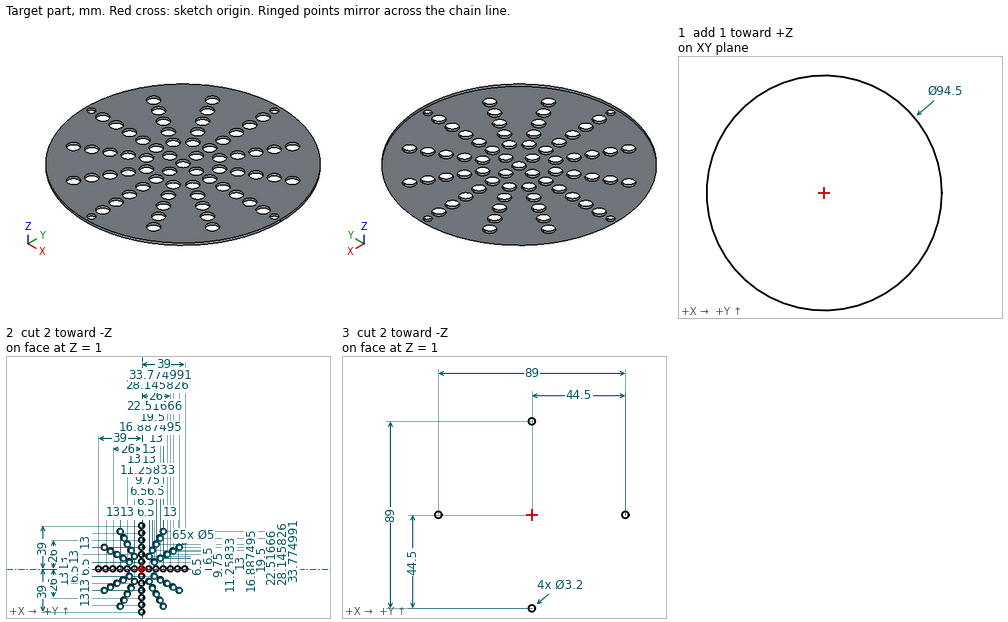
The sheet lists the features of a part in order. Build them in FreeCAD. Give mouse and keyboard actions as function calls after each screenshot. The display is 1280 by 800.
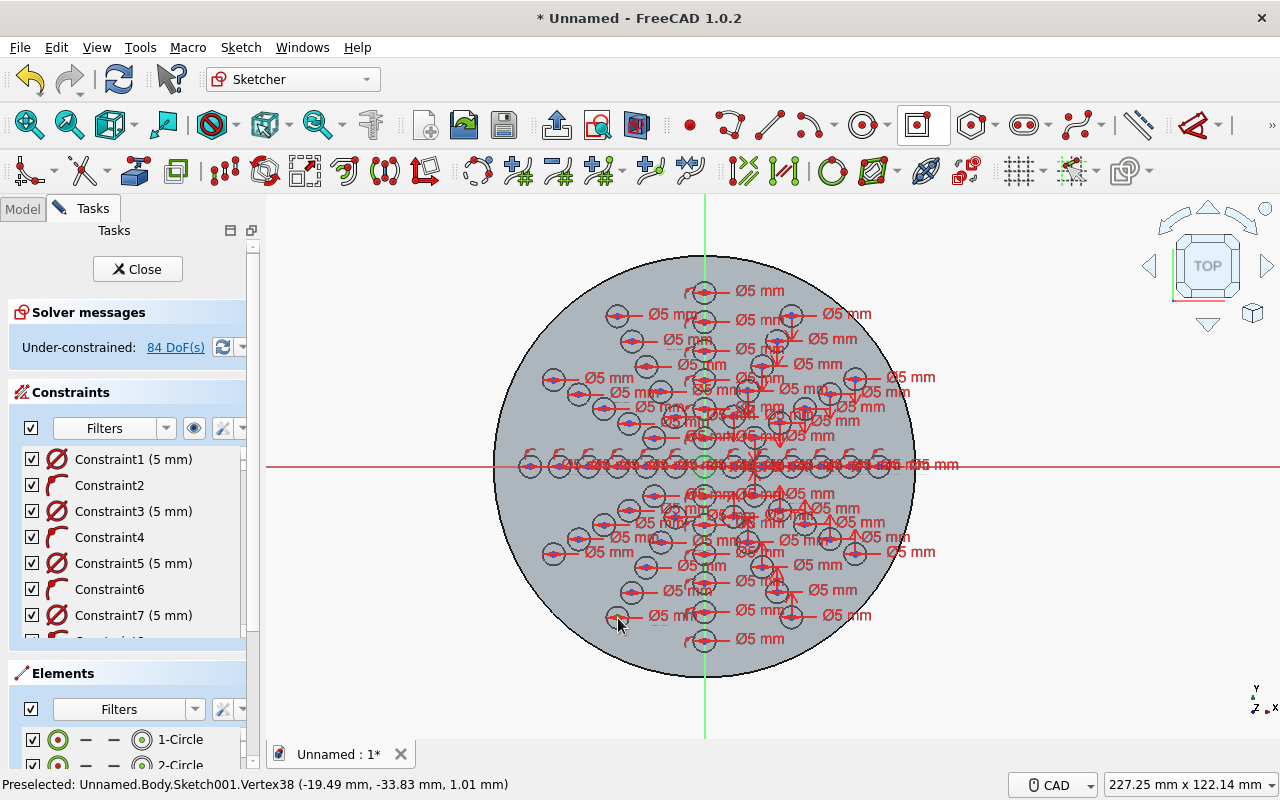
click(705, 257)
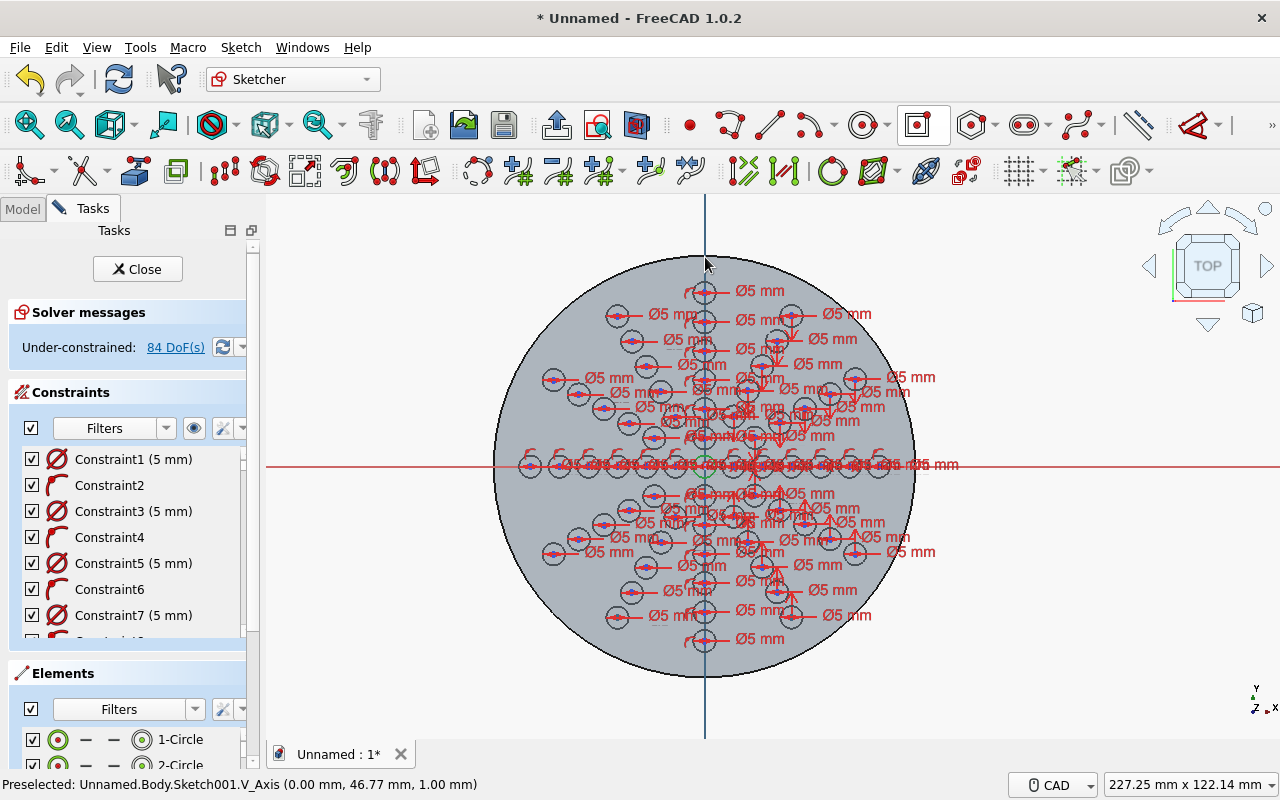
key(s)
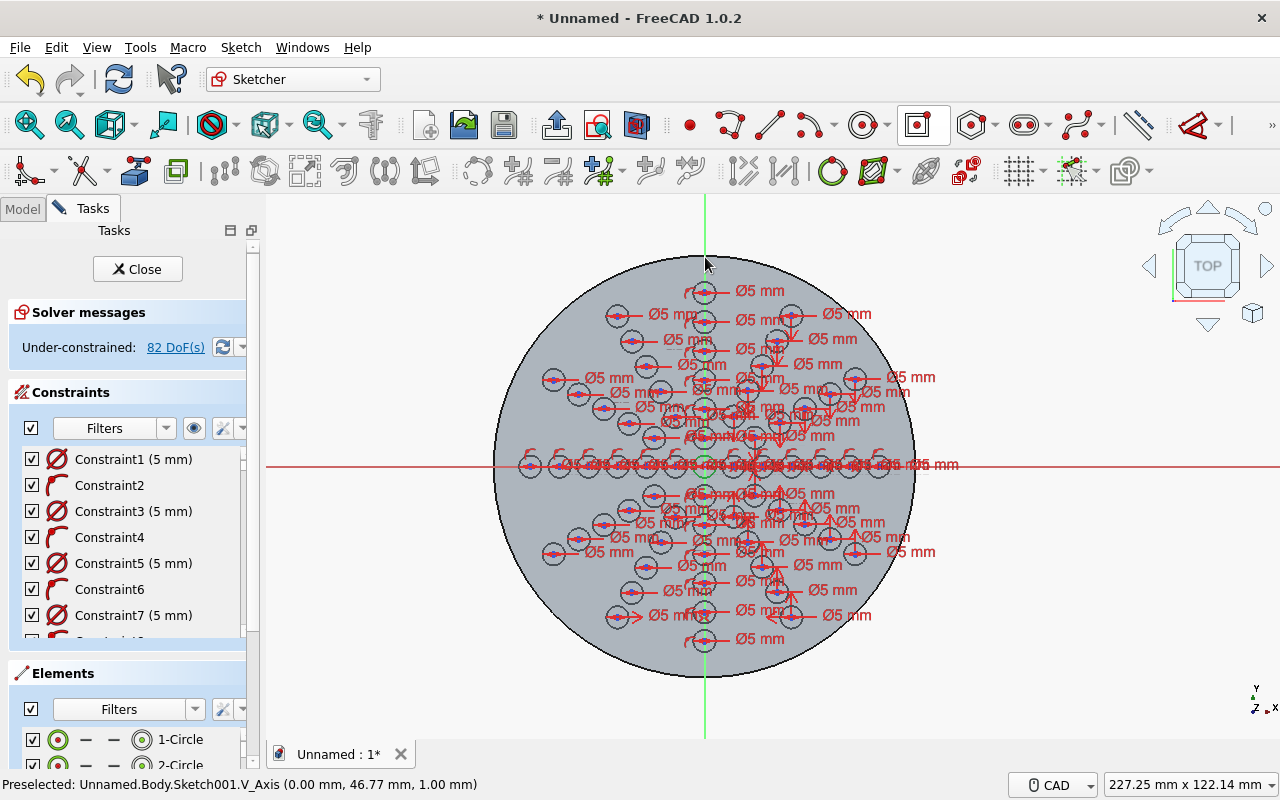
click(777, 592)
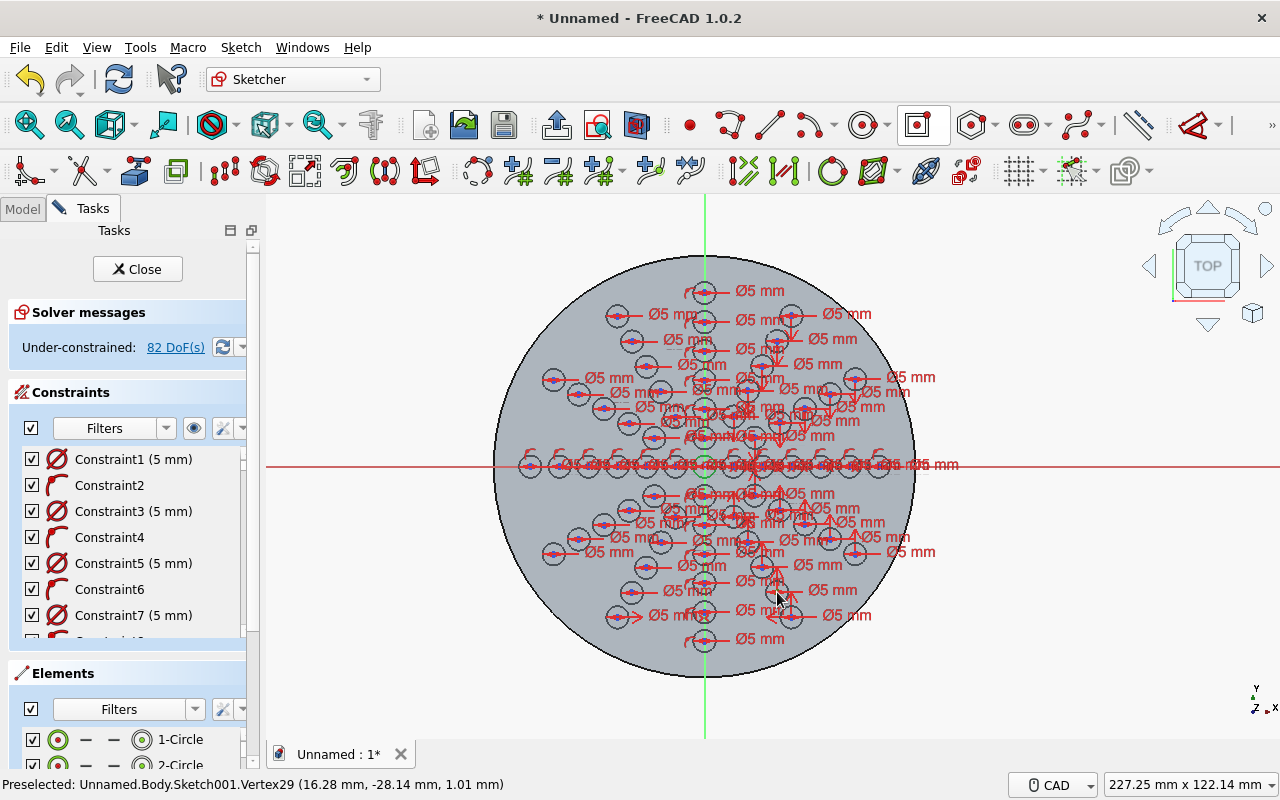
click(632, 593)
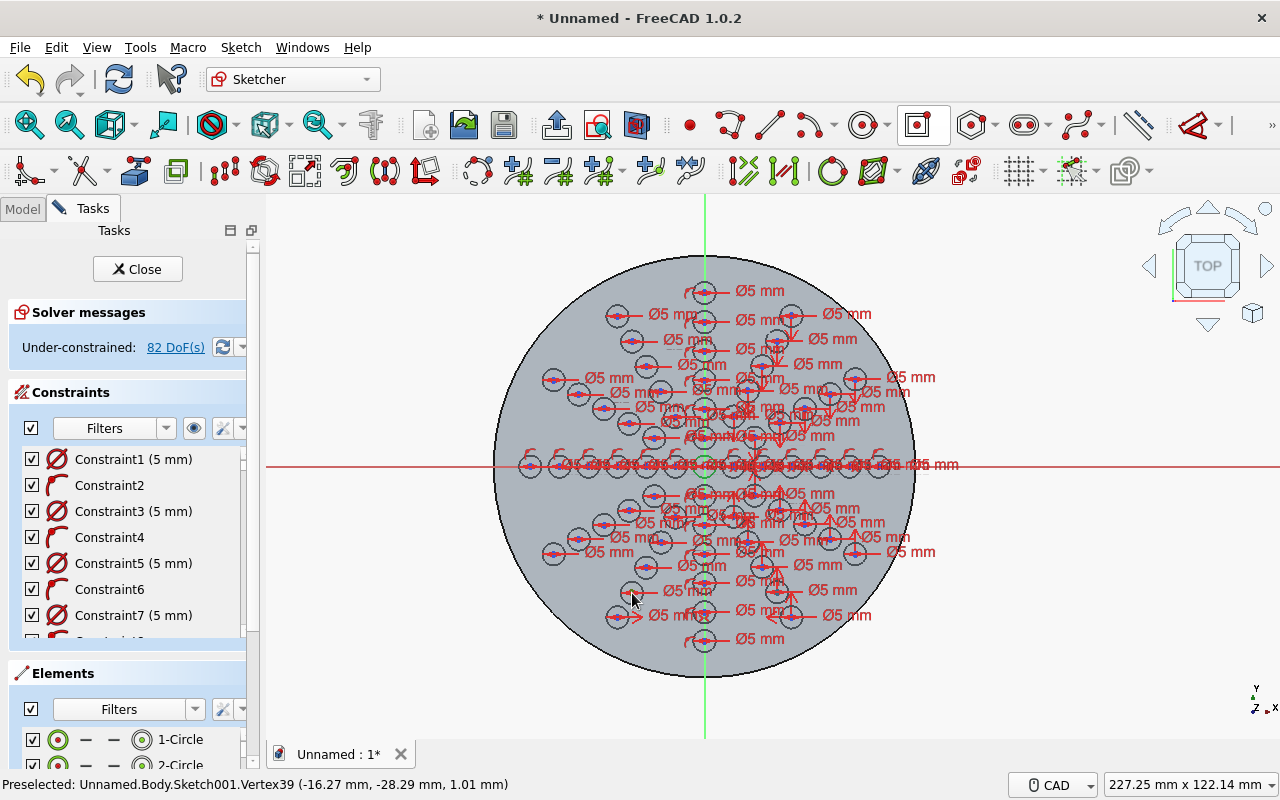
click(705, 257)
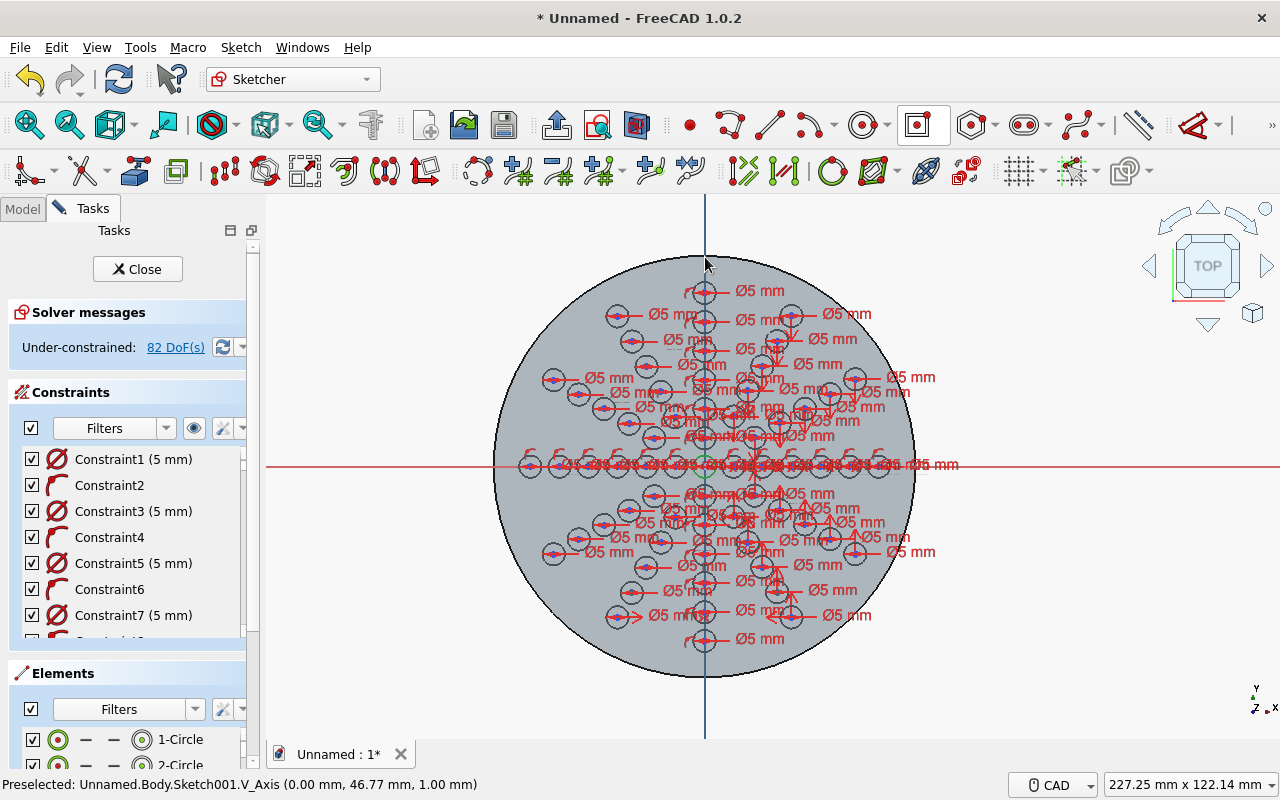
key(s)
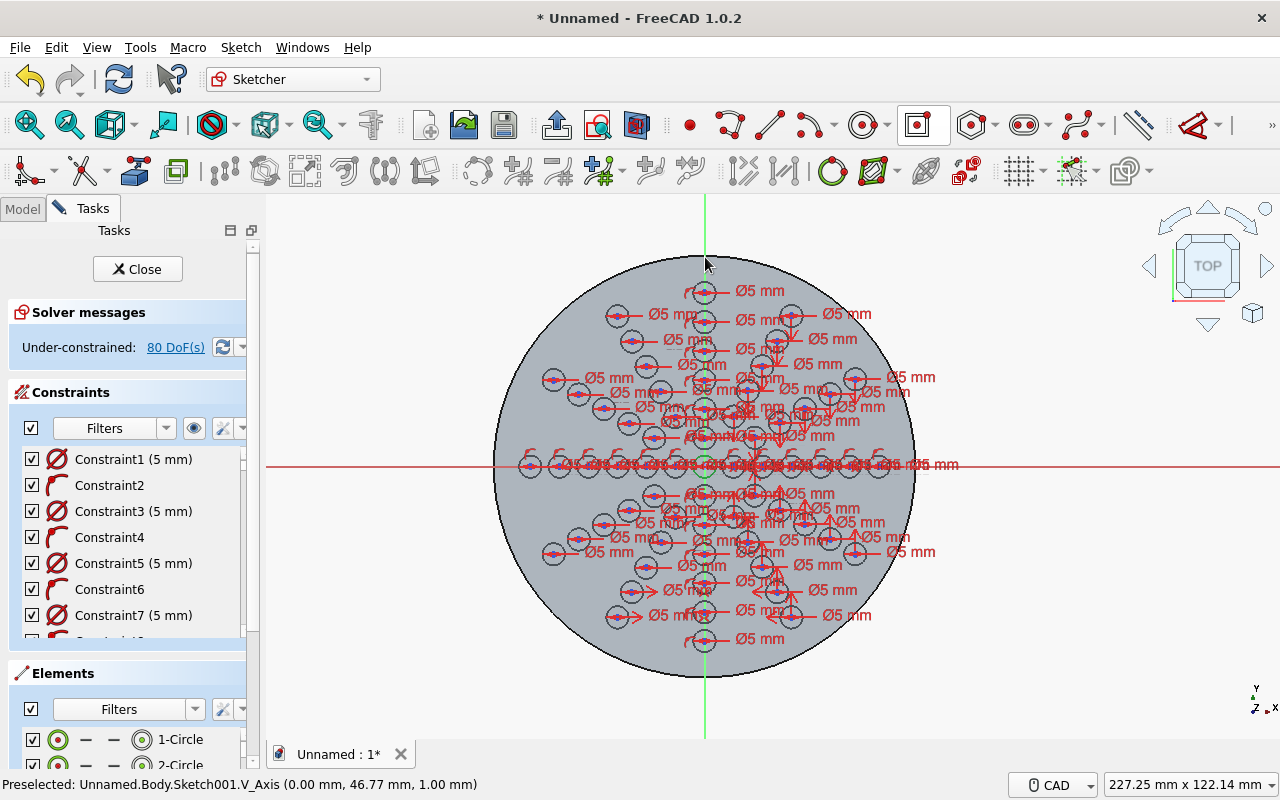
click(762, 567)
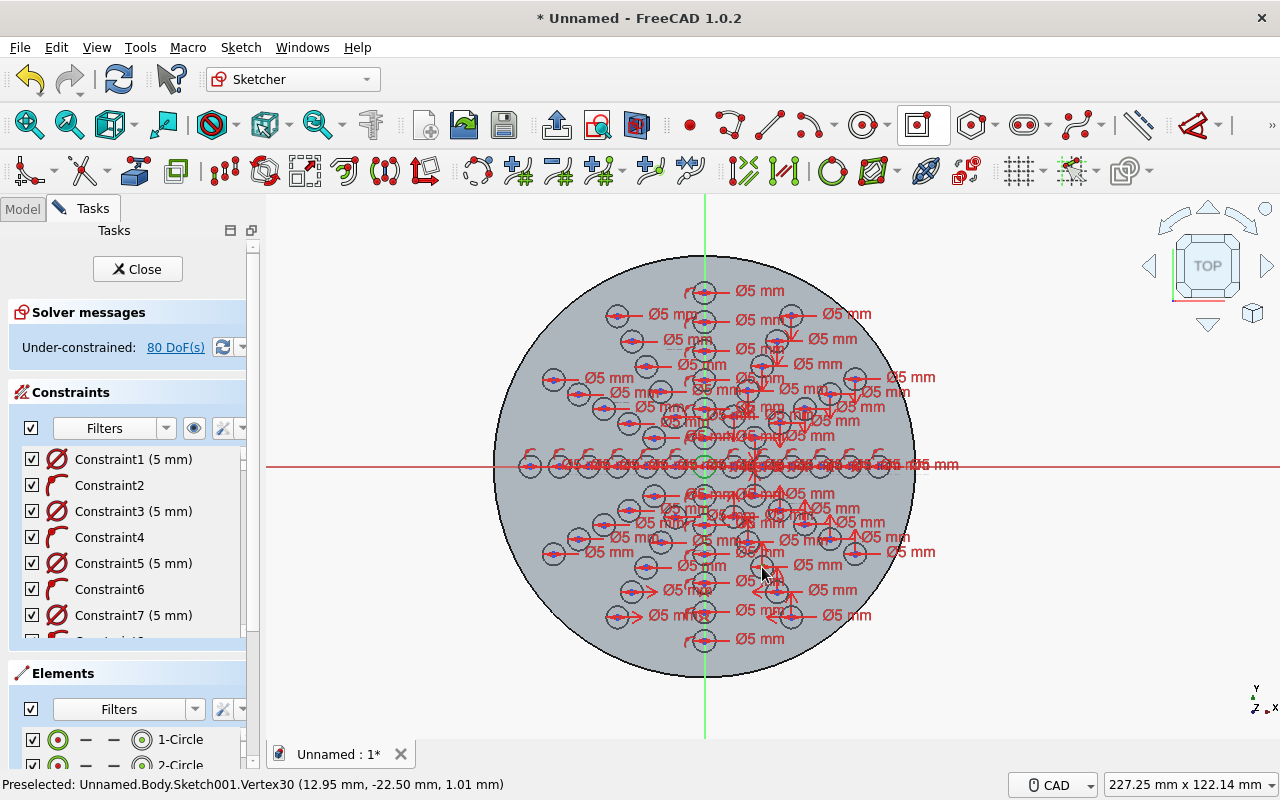
click(646, 568)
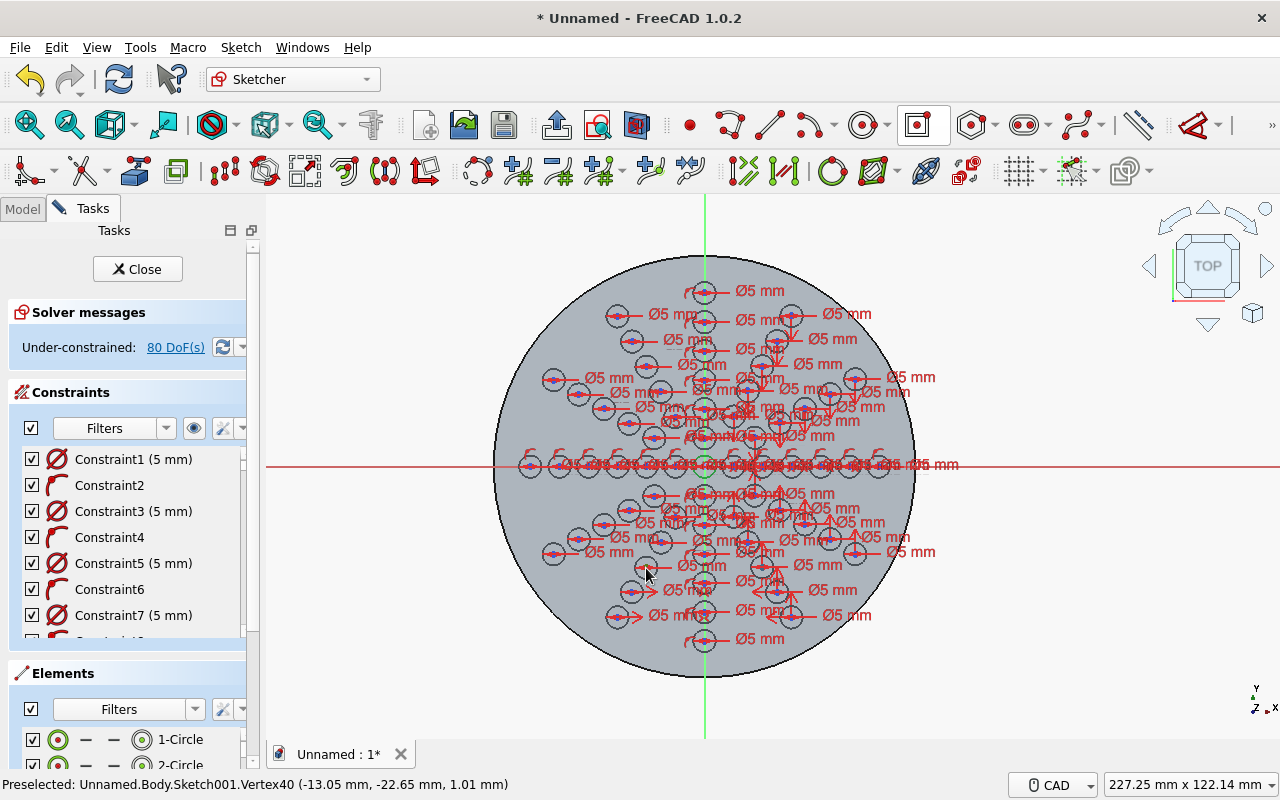
click(705, 257)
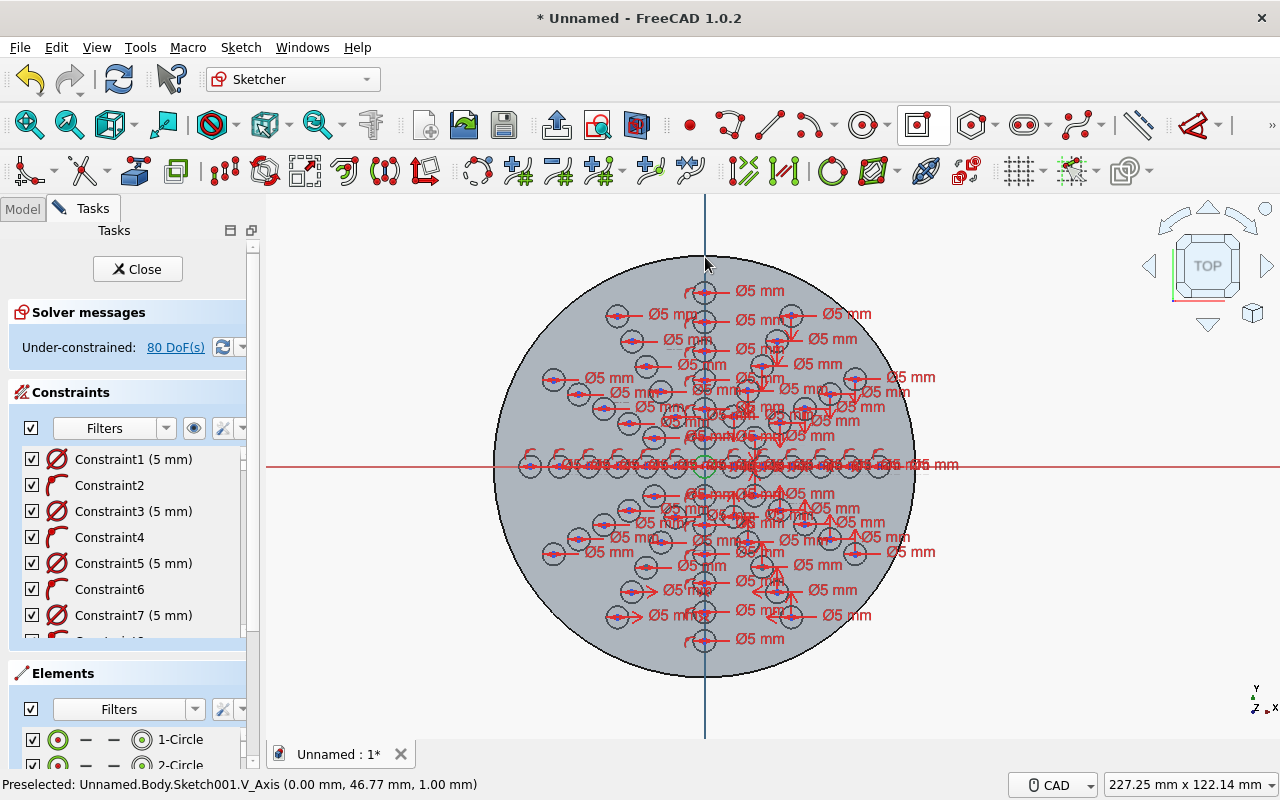
key(s)